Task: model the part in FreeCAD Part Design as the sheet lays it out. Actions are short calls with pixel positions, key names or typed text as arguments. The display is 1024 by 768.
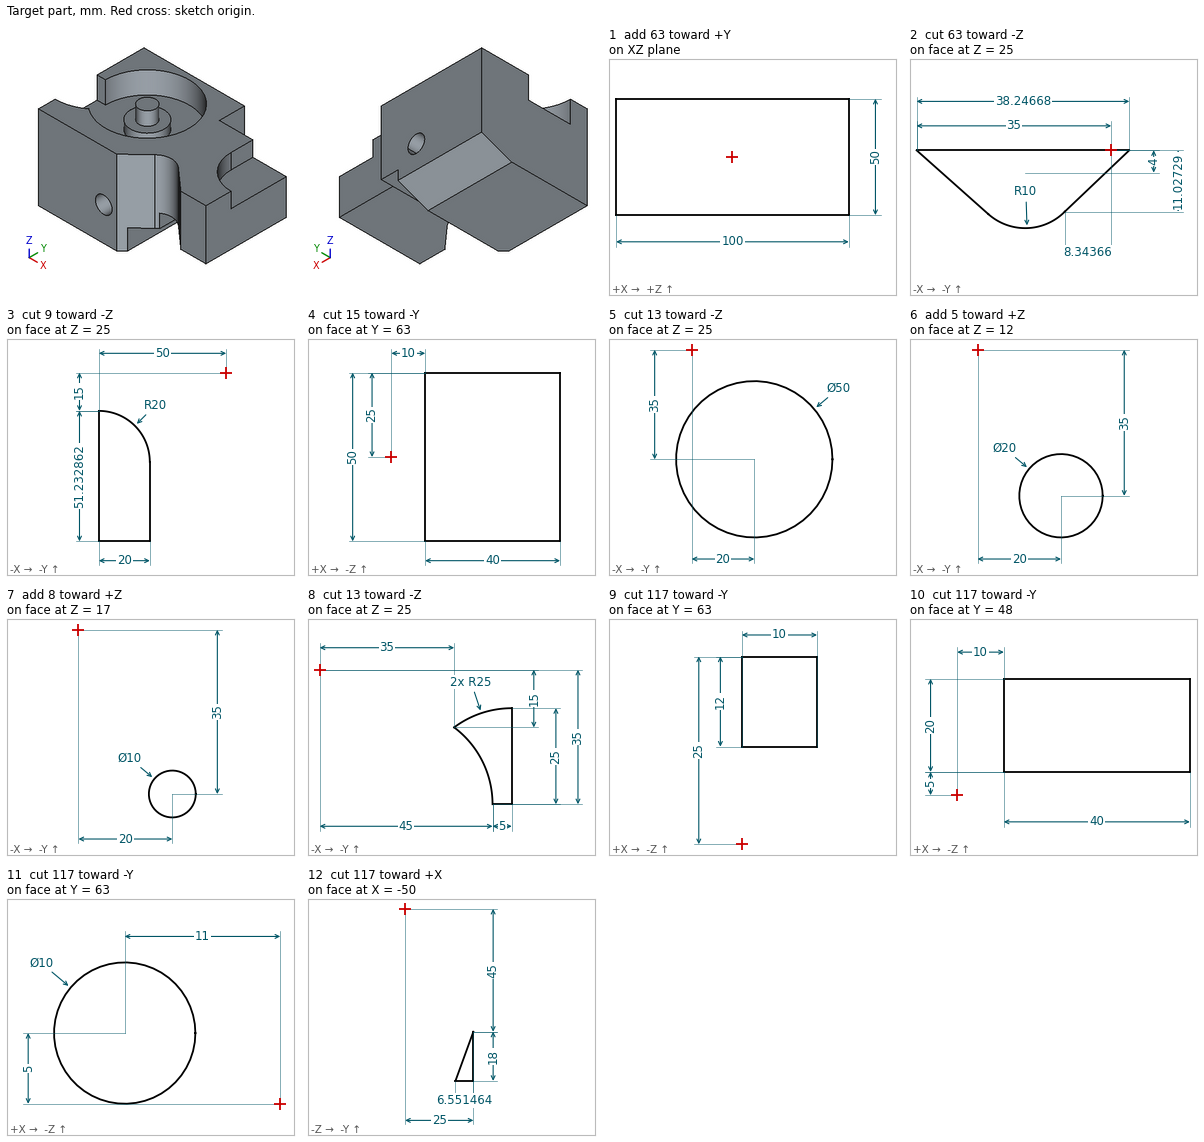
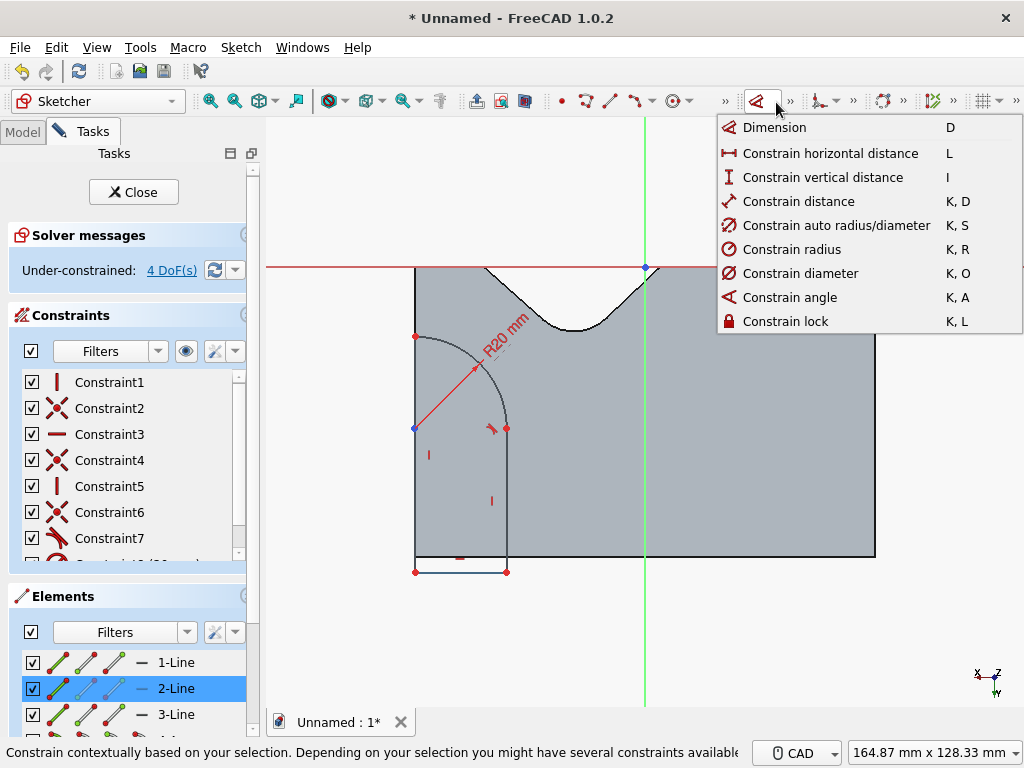
click(870, 153)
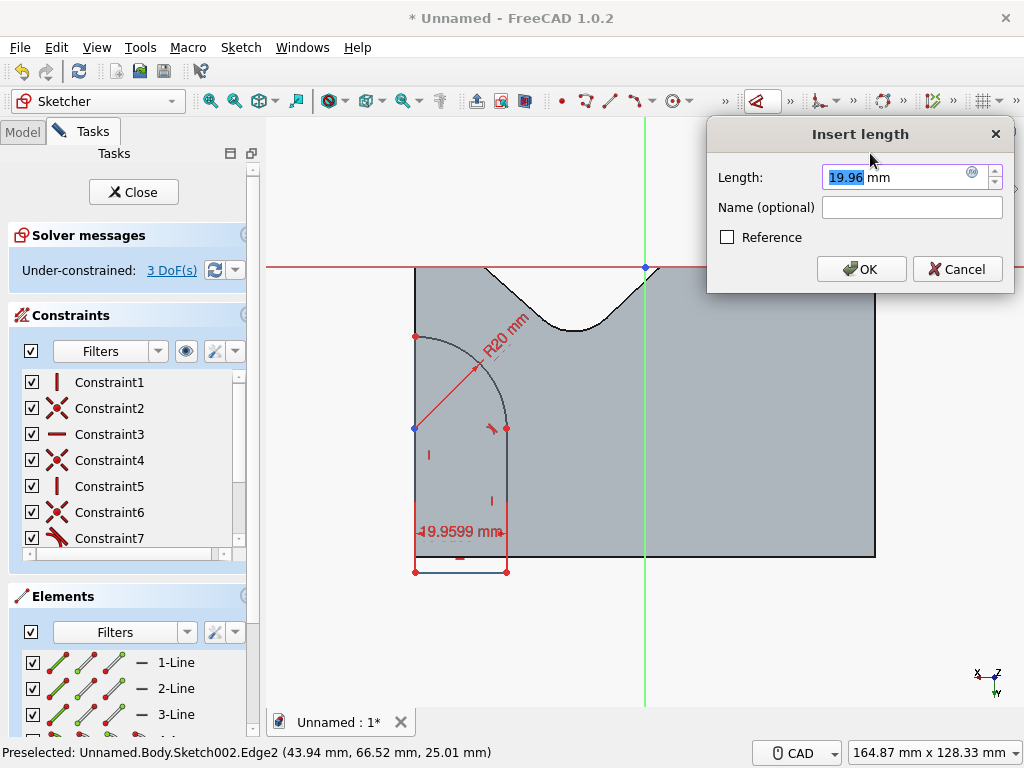
text(20)
key(Return)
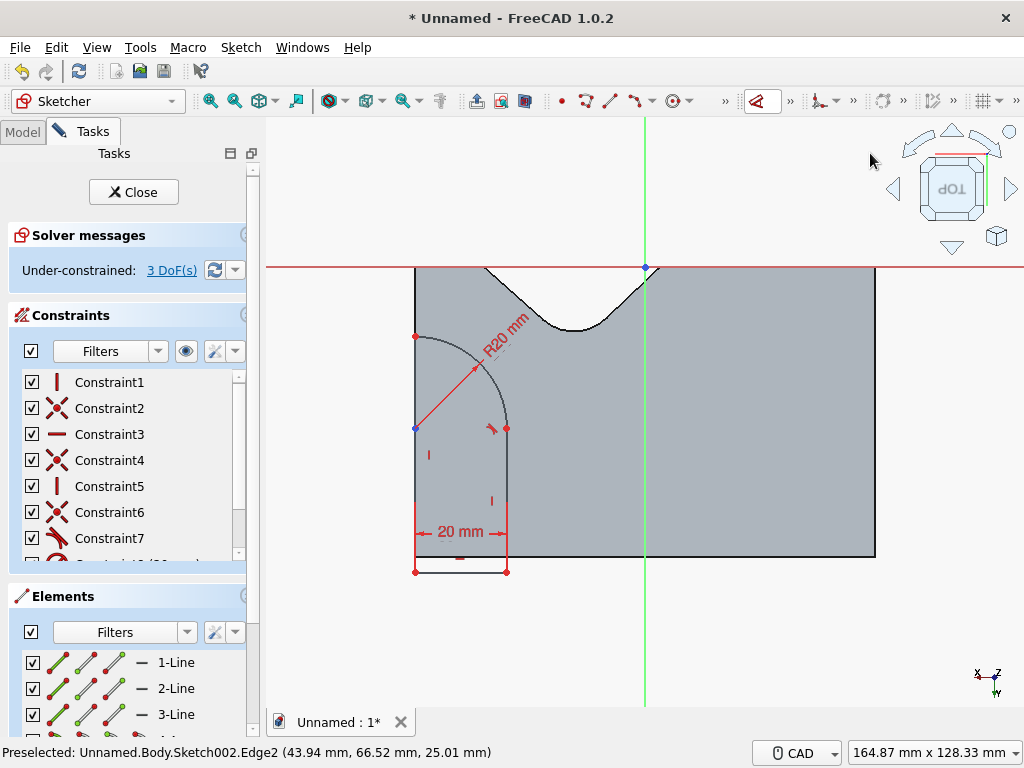
click(415, 337)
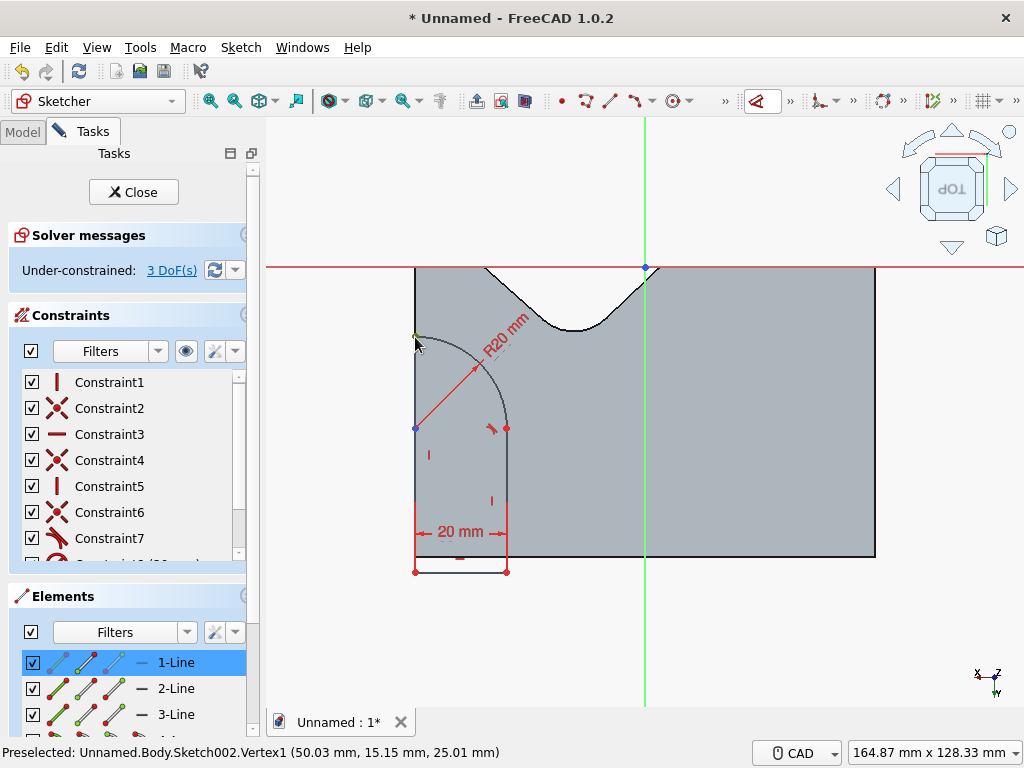
key(l)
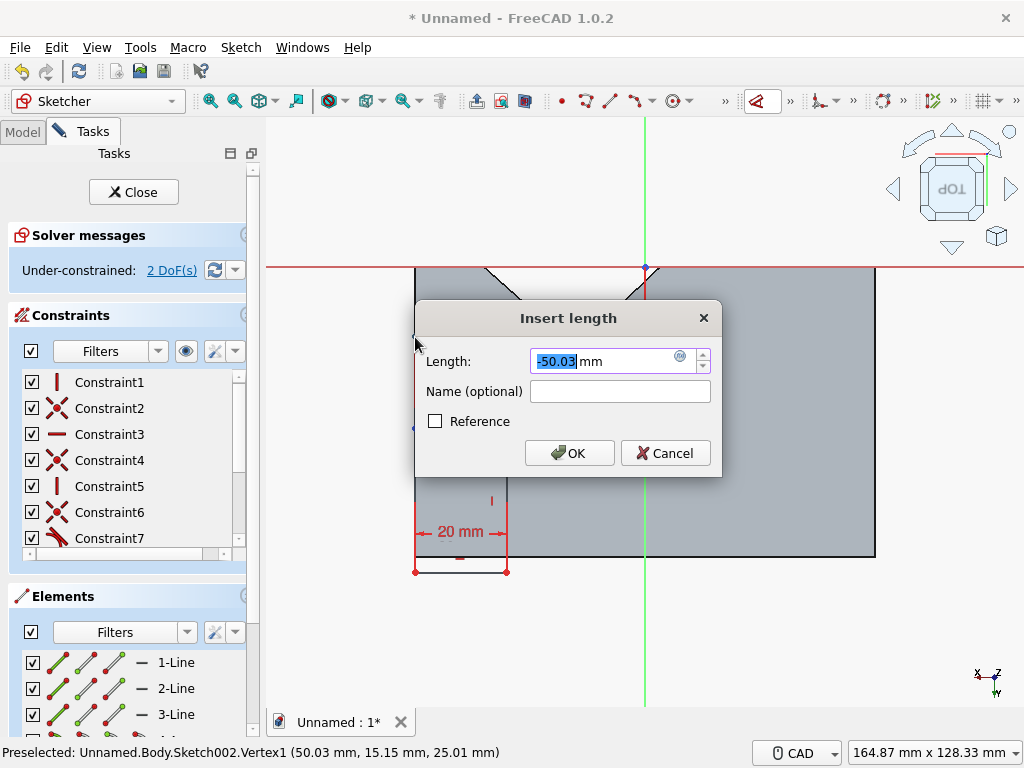
text(-50)
key(Return)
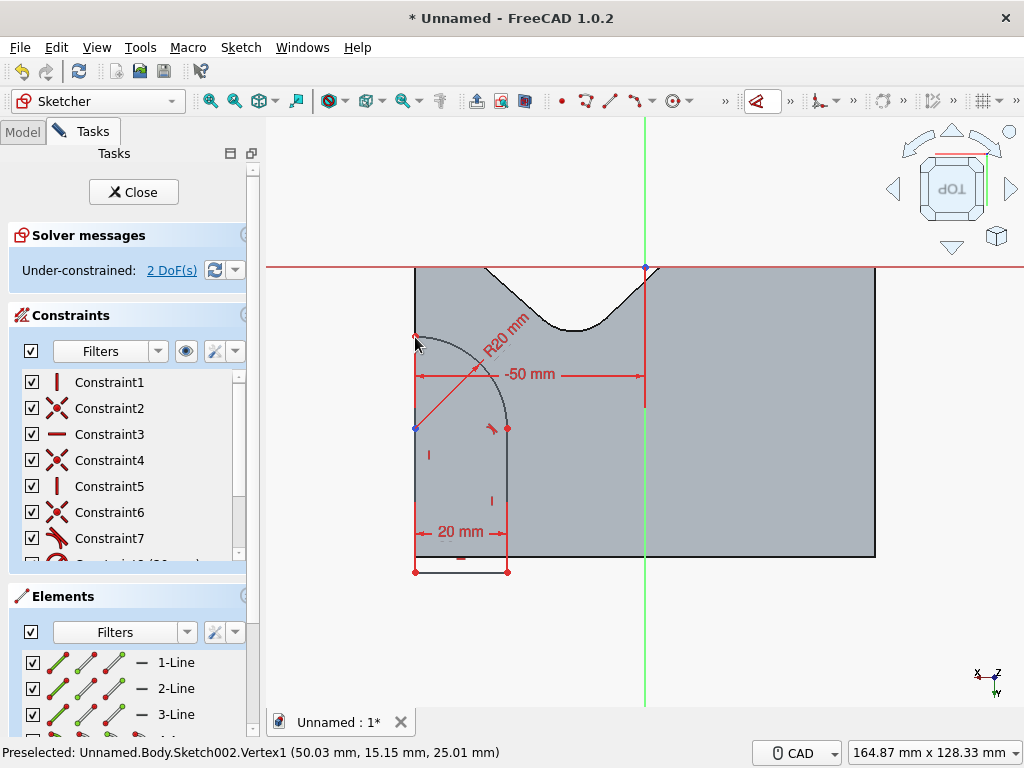
click(415, 337)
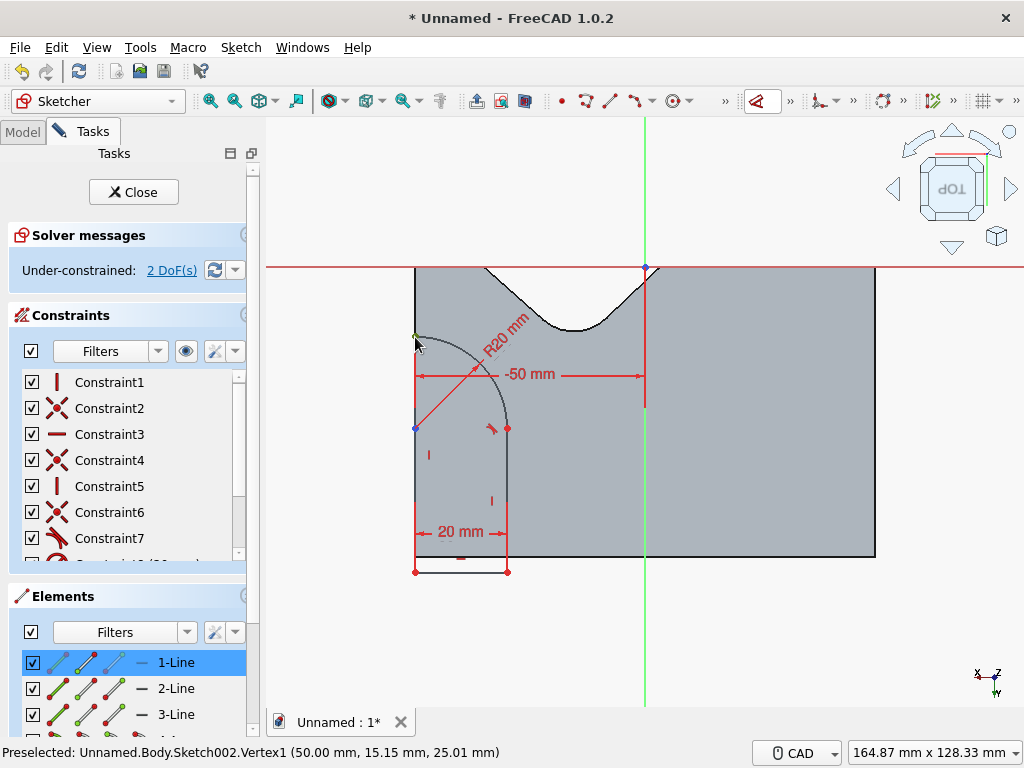
click(776, 102)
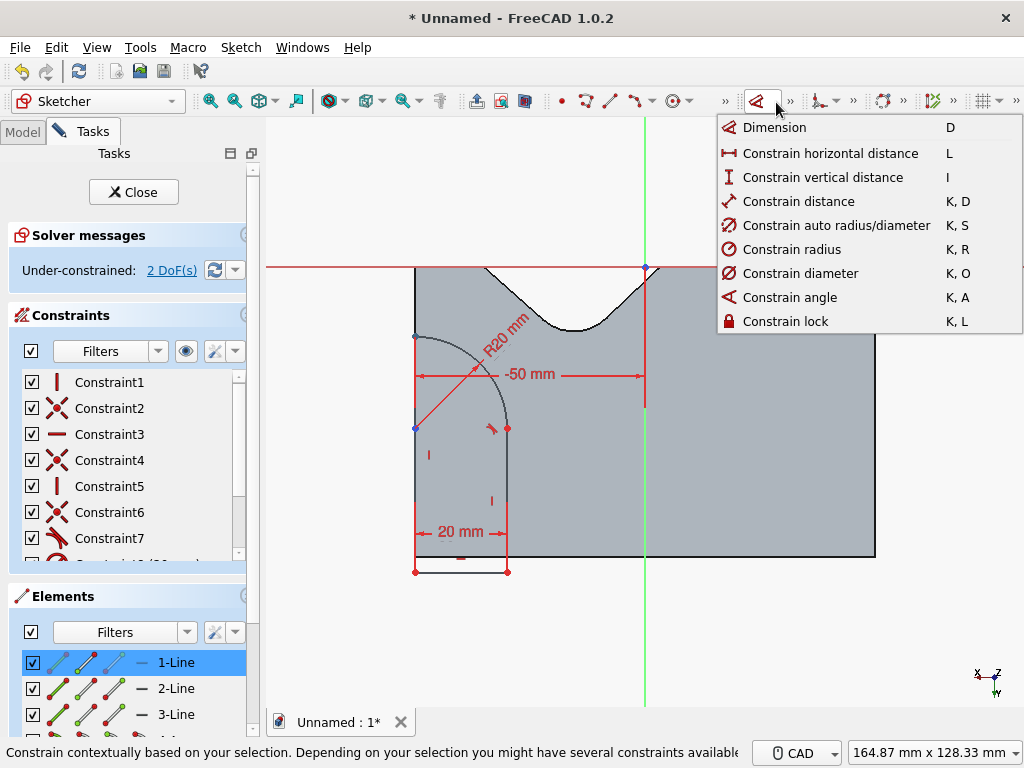
click(870, 177)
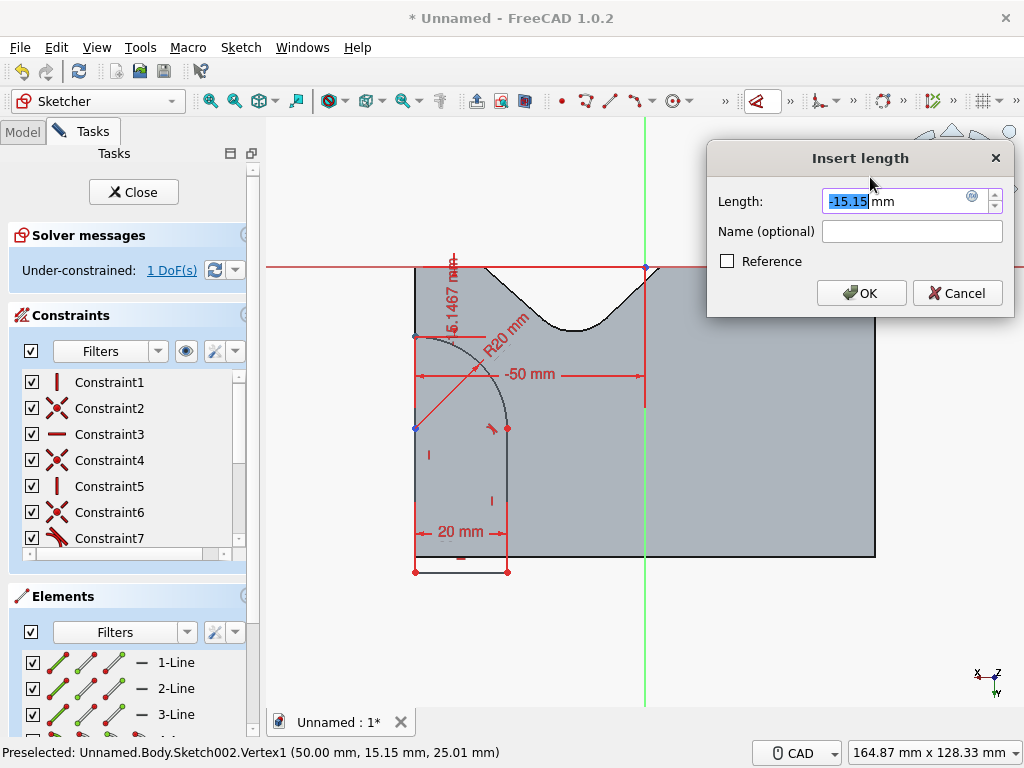
text(-15)
key(Return)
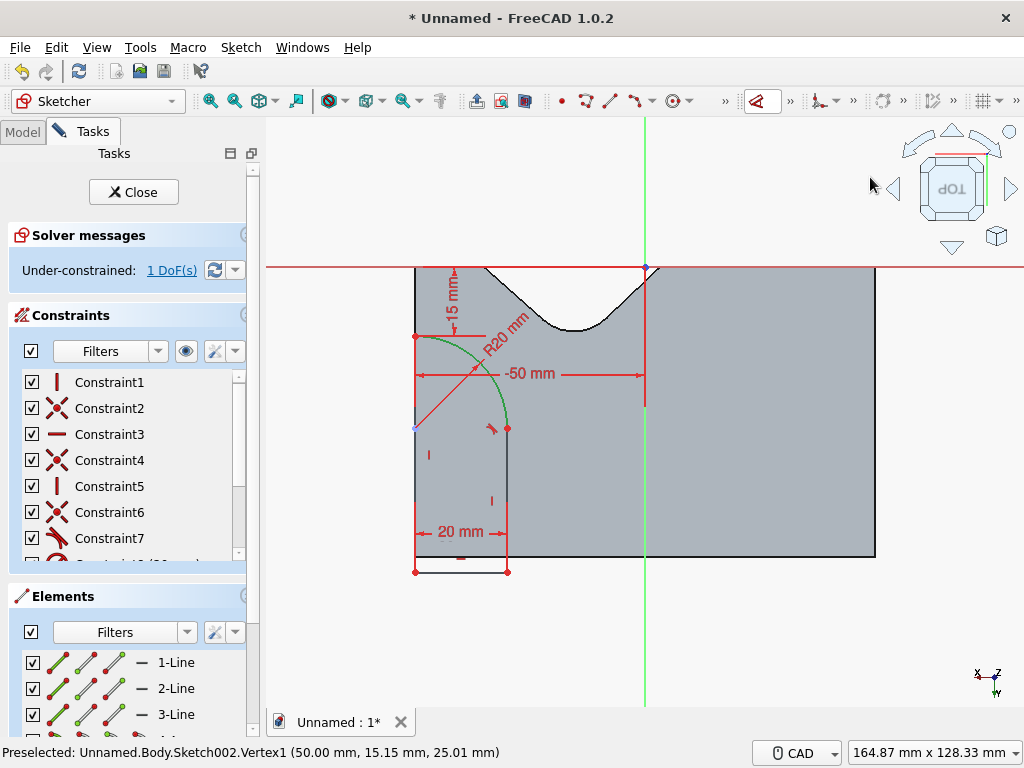
click(415, 407)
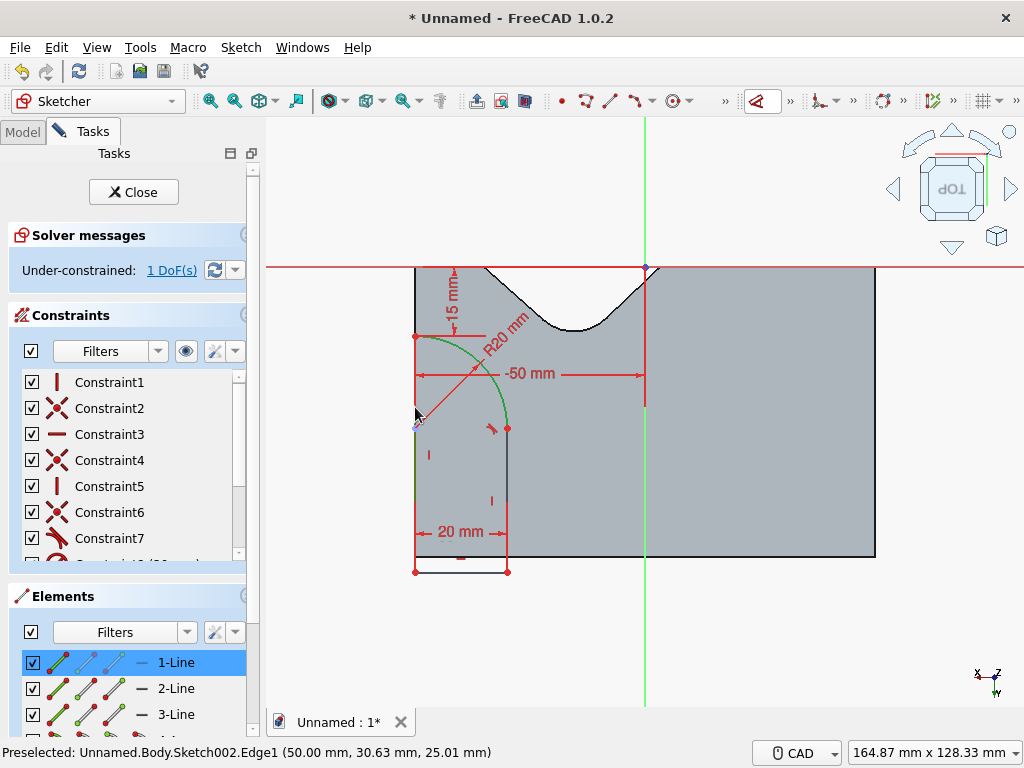
click(776, 102)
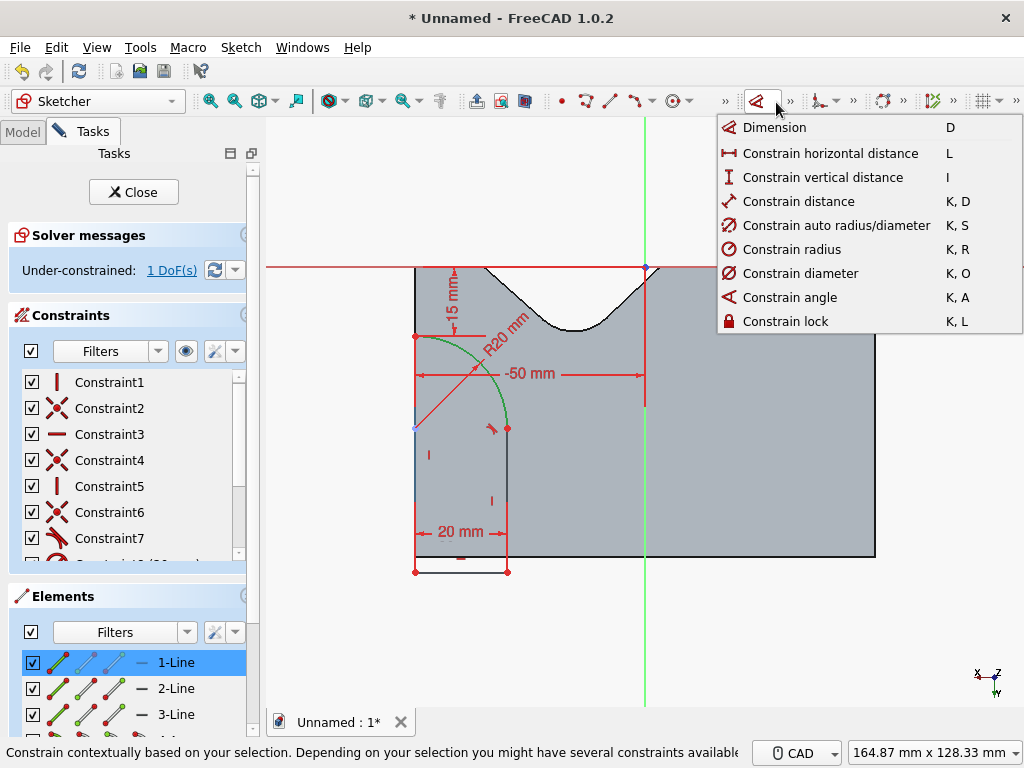
click(870, 177)